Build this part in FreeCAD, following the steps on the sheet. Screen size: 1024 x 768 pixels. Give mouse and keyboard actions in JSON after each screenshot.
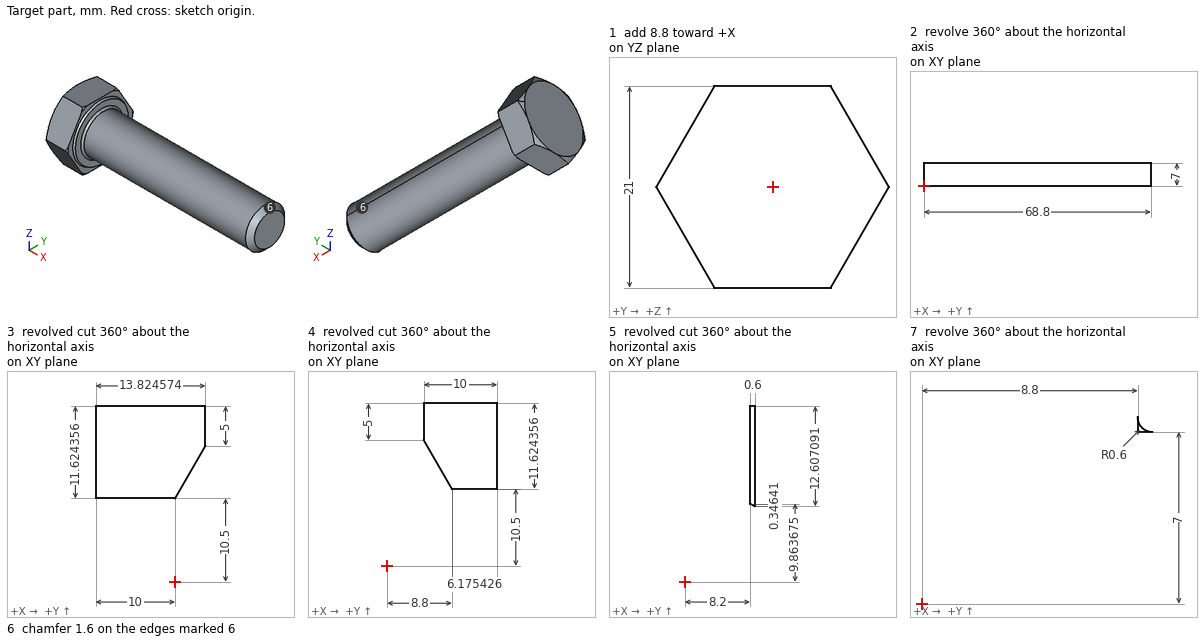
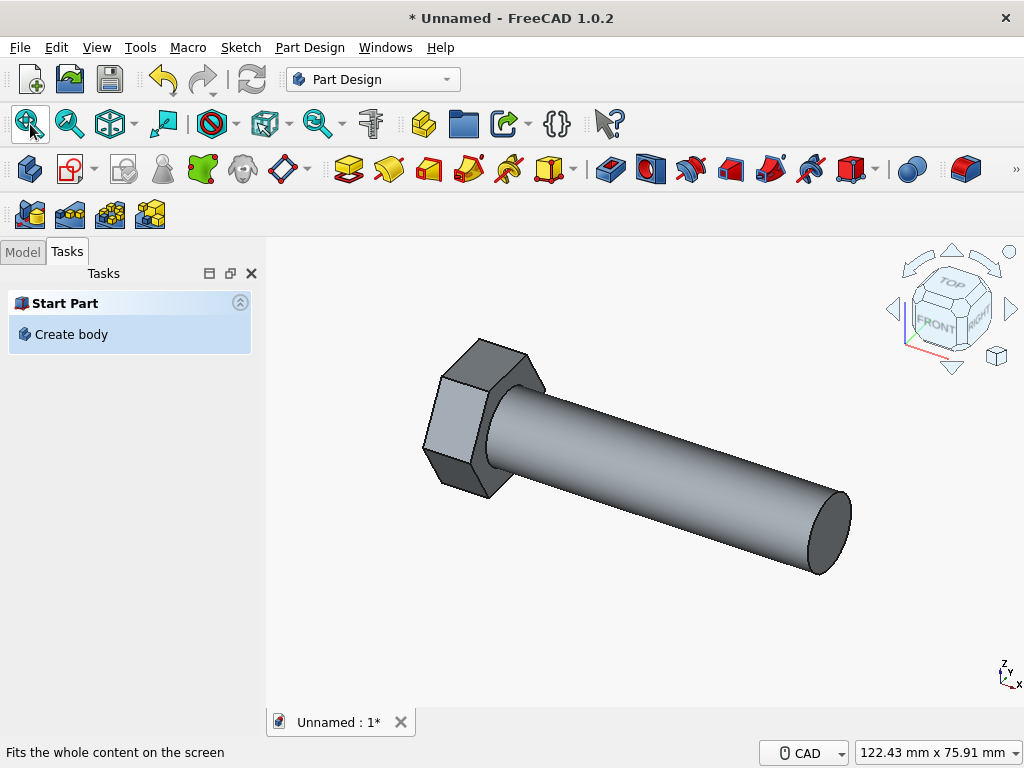
{"action": "left_click", "coordinate": [70, 170]}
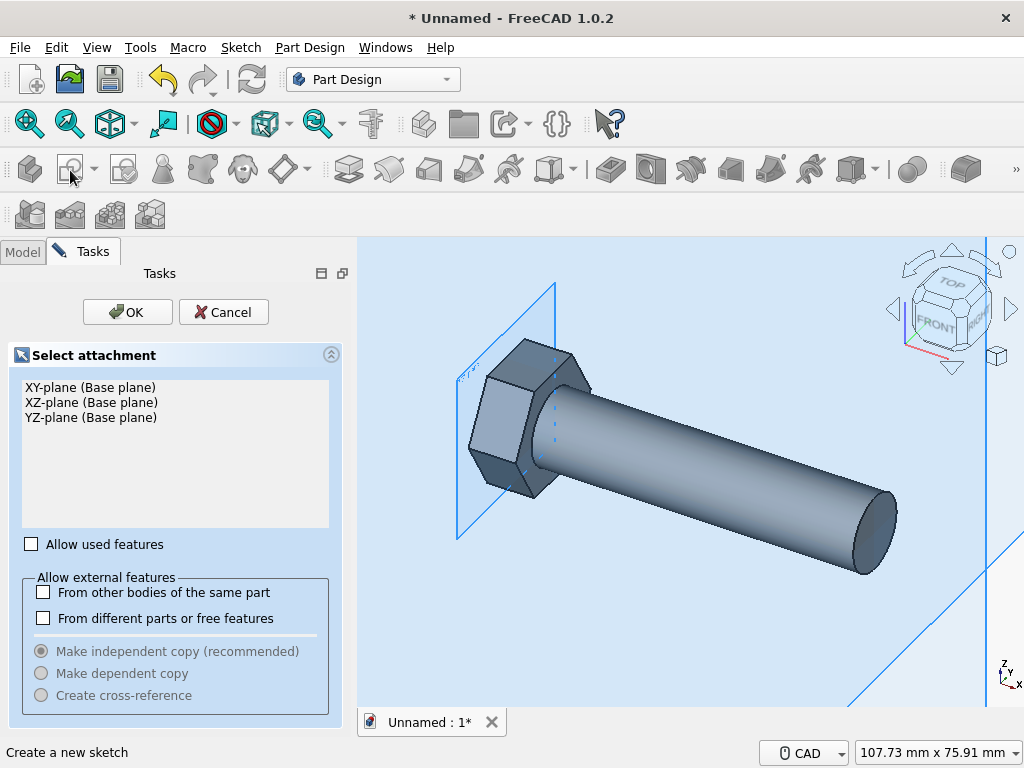
{"action": "left_click", "coordinate": [82, 388]}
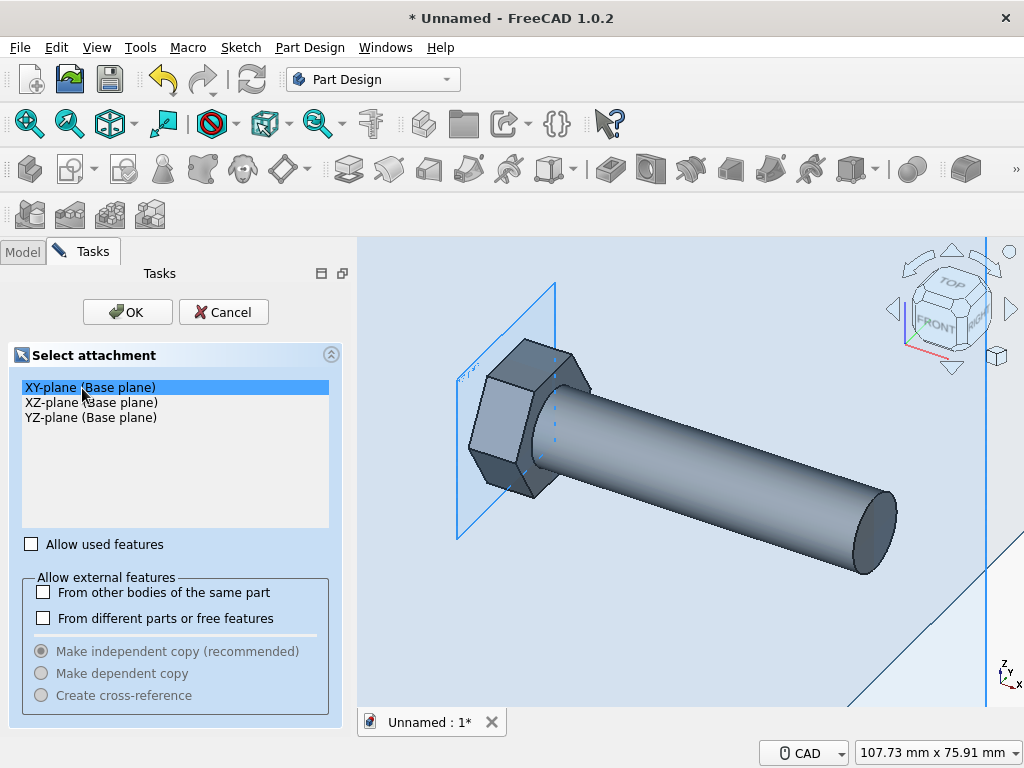
{"action": "left_click", "coordinate": [128, 312]}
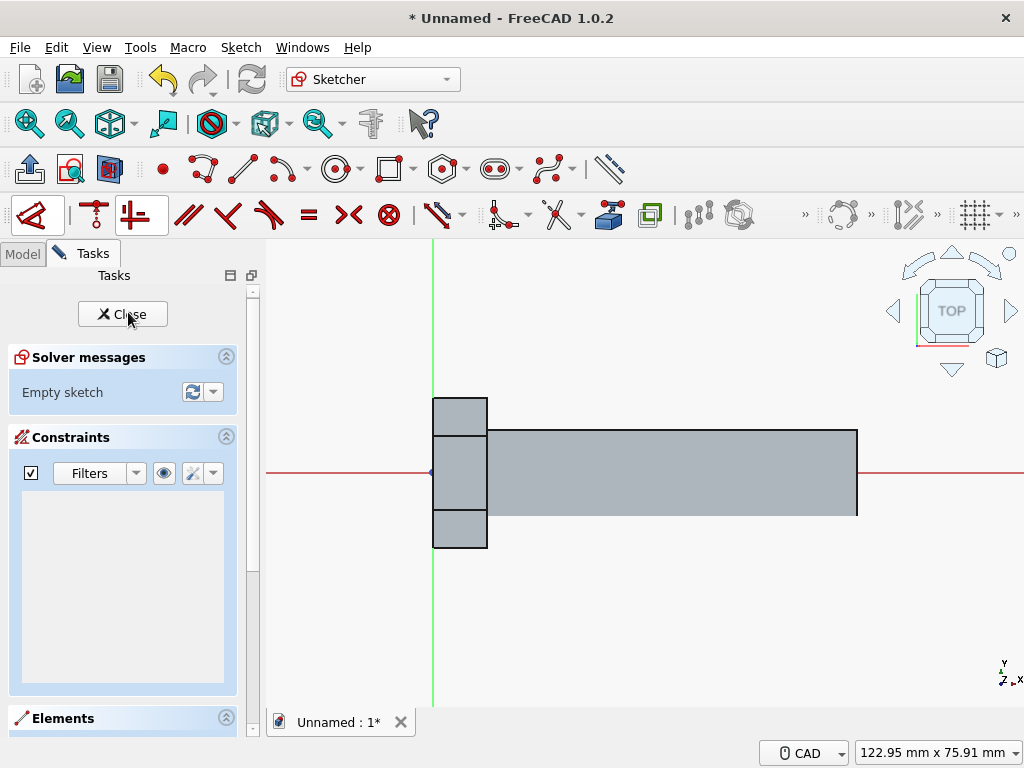
{"action": "left_click", "coordinate": [110, 170]}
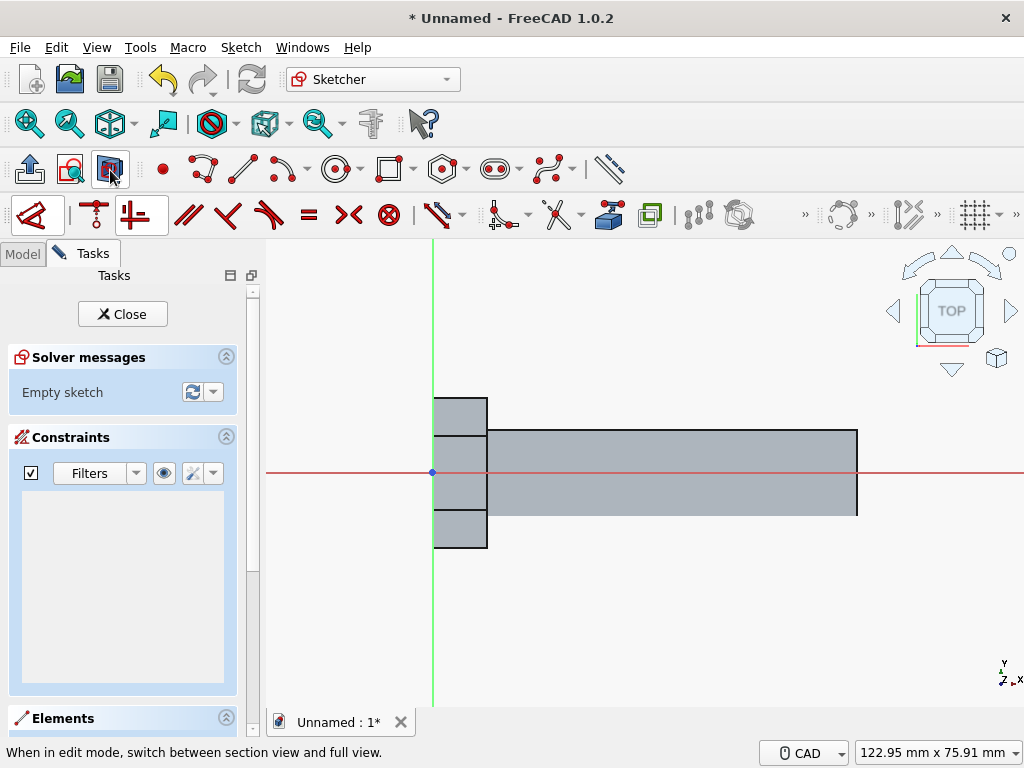
{"action": "scroll", "coordinate": [294, 349], "scroll_direction": "up", "scroll_amount": 4}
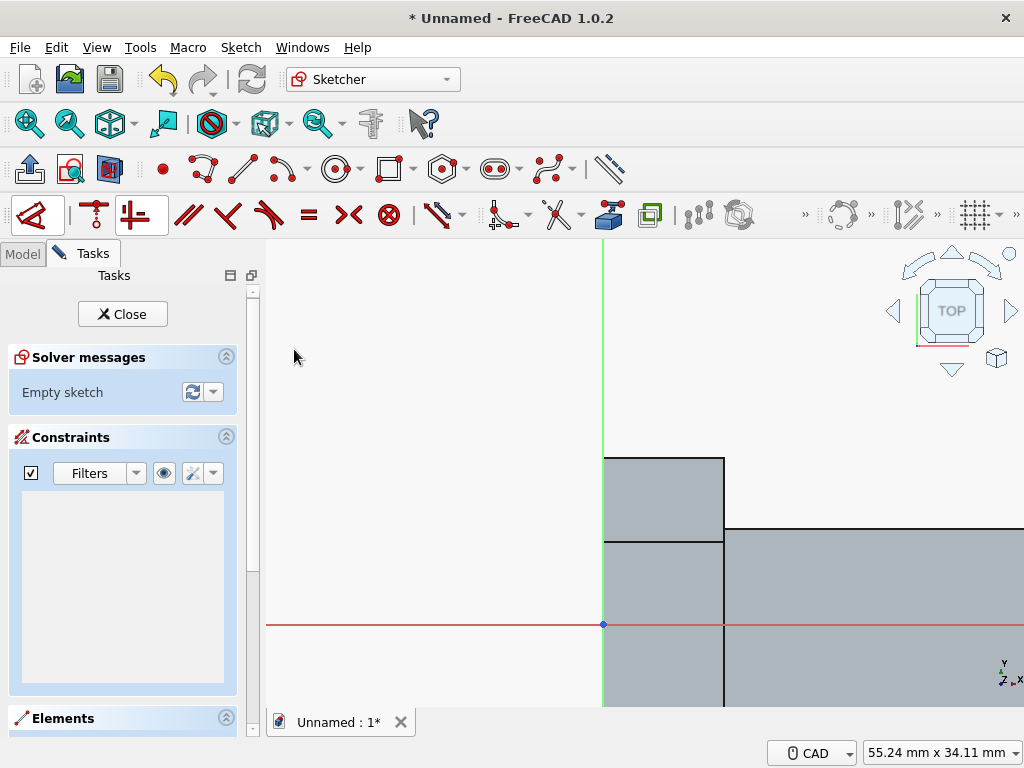
{"action": "left_click", "coordinate": [204, 170]}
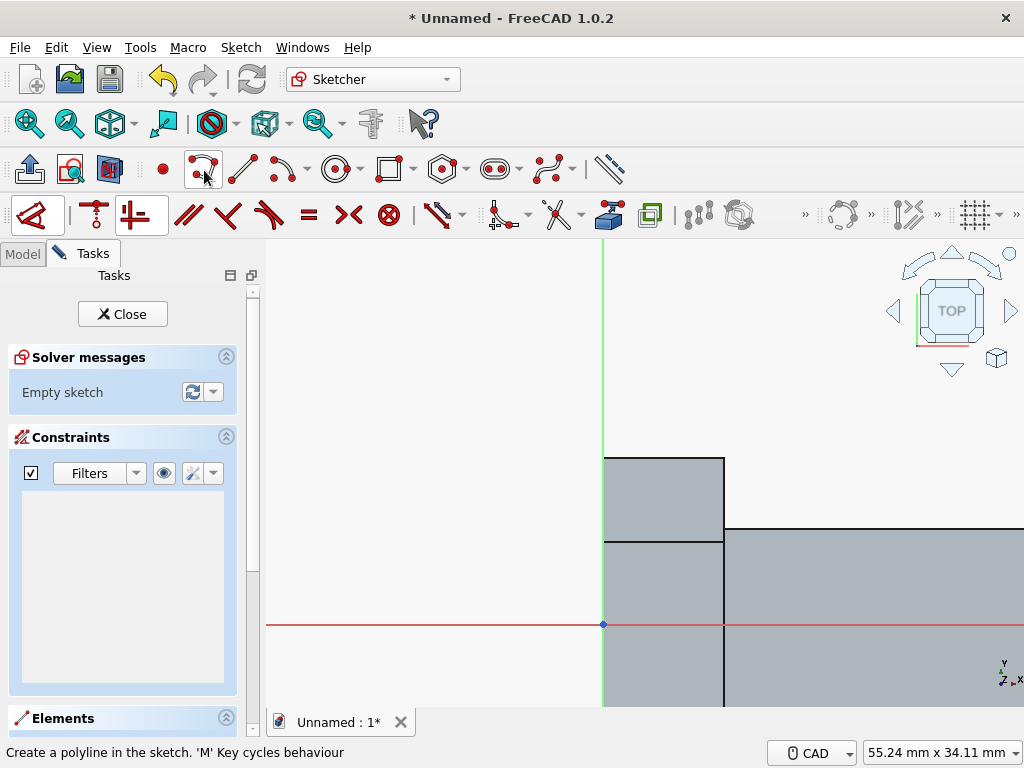
{"action": "left_click", "coordinate": [603, 481]}
{"action": "left_click", "coordinate": [656, 390]}
{"action": "left_click", "coordinate": [656, 321]}
{"action": "left_click", "coordinate": [466, 321]}
{"action": "left_click", "coordinate": [466, 481]}
{"action": "left_click", "coordinate": [603, 482]}
{"action": "key", "text": "Escape"}
{"action": "key", "text": "Escape"}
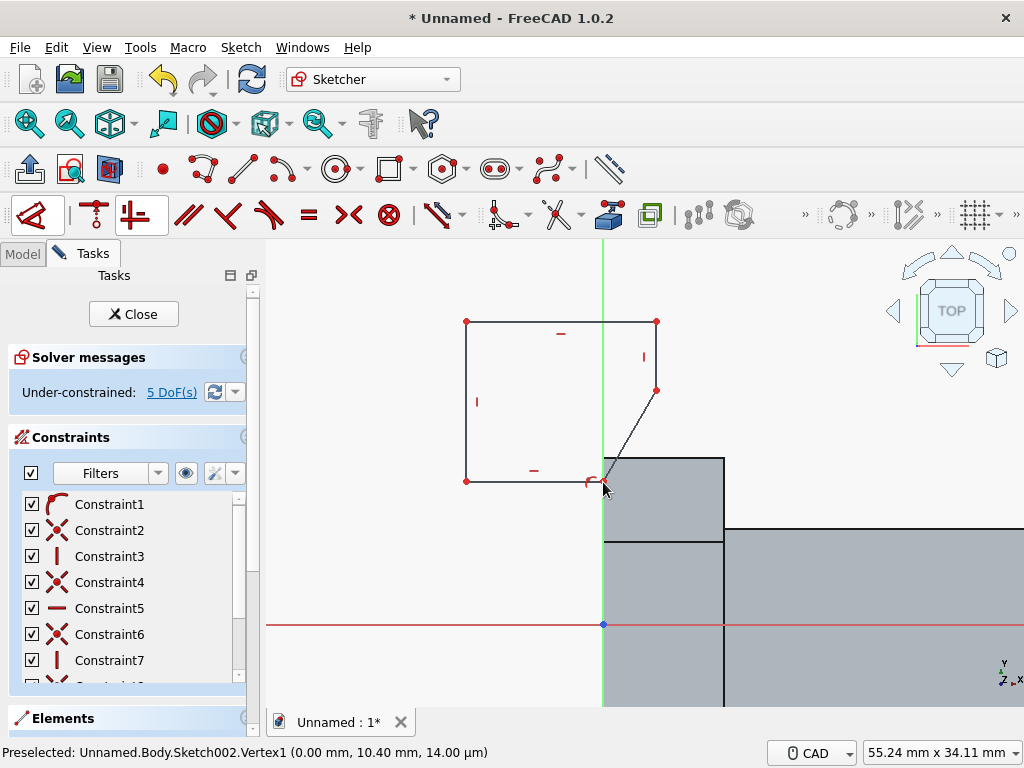
{"action": "left_click", "coordinate": [656, 370]}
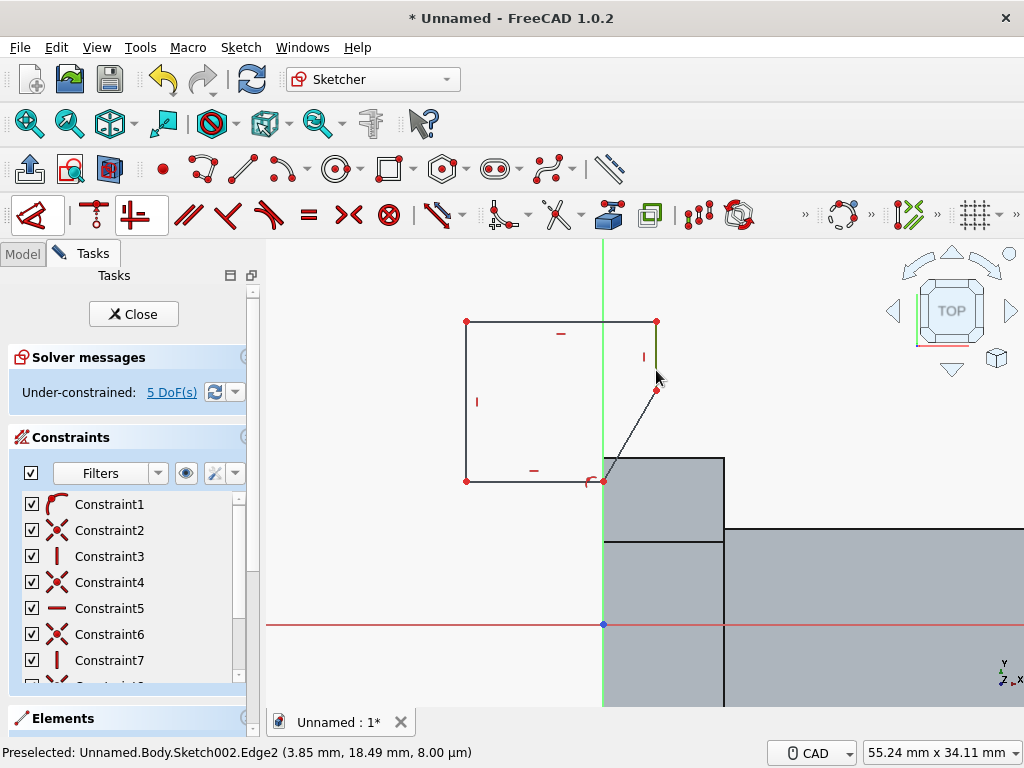
{"action": "left_click", "coordinate": [58, 216]}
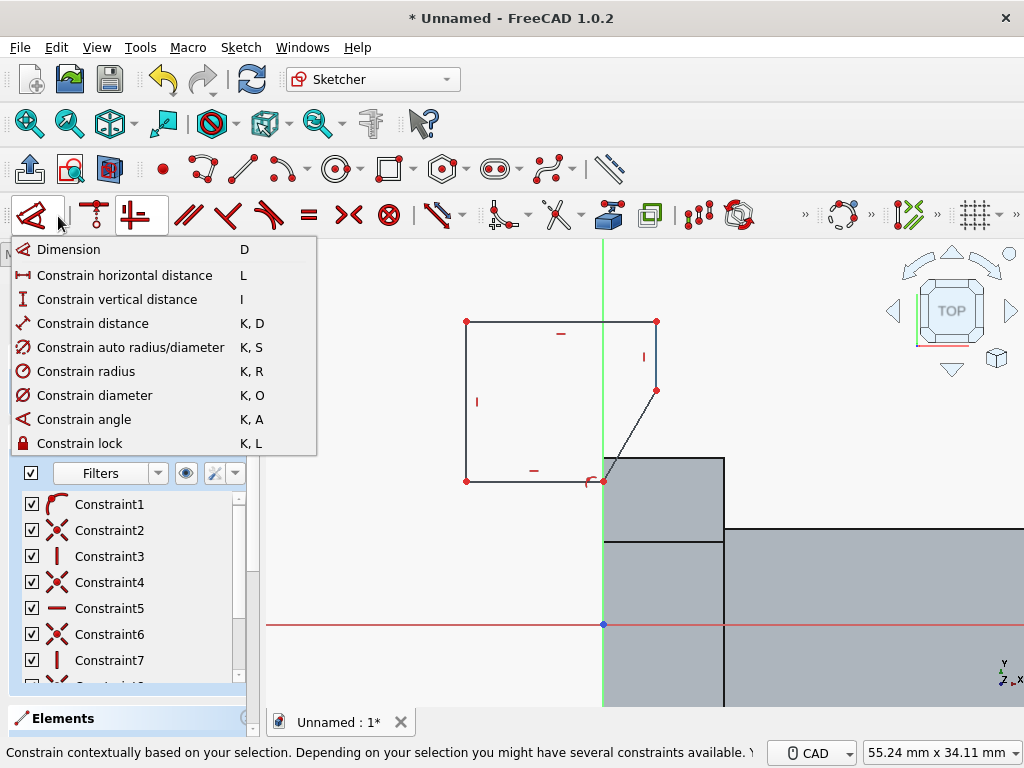
{"action": "left_click", "coordinate": [164, 299]}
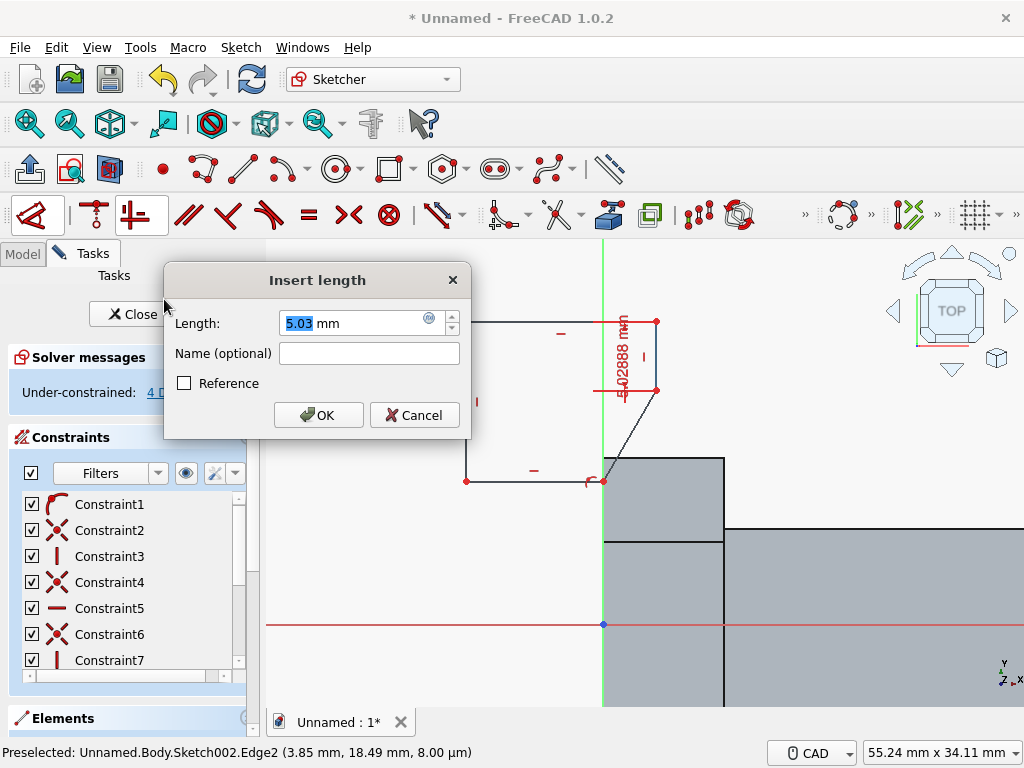
{"action": "type", "text": "5"}
{"action": "key", "text": "Return"}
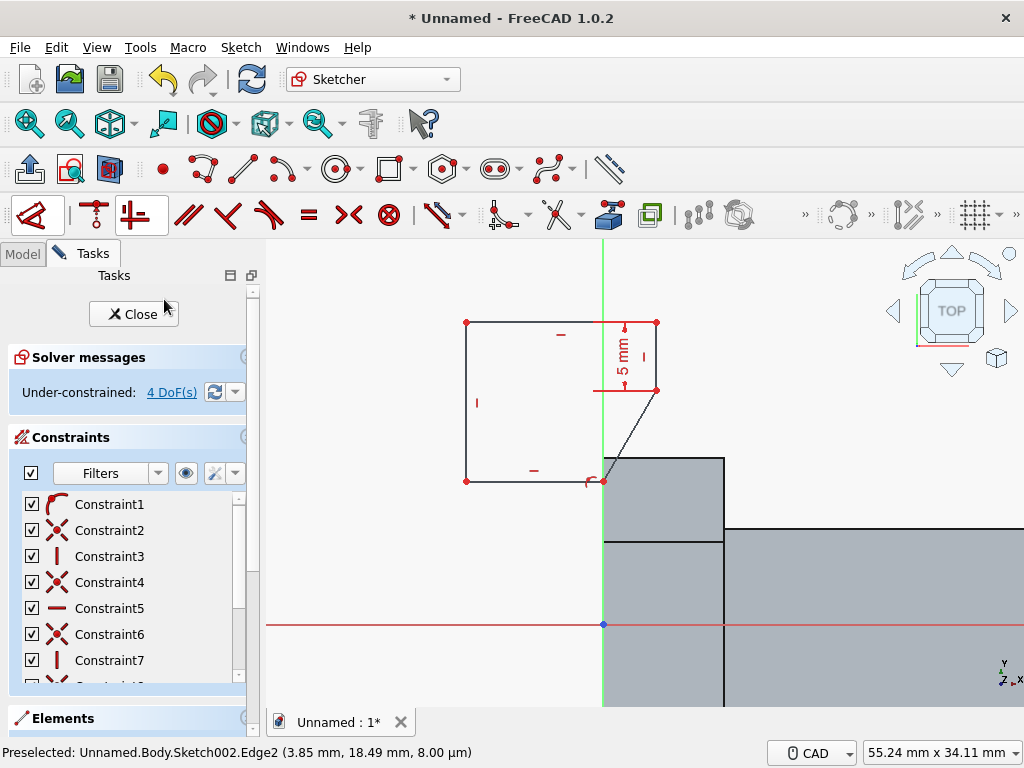
{"action": "left_click", "coordinate": [507, 482]}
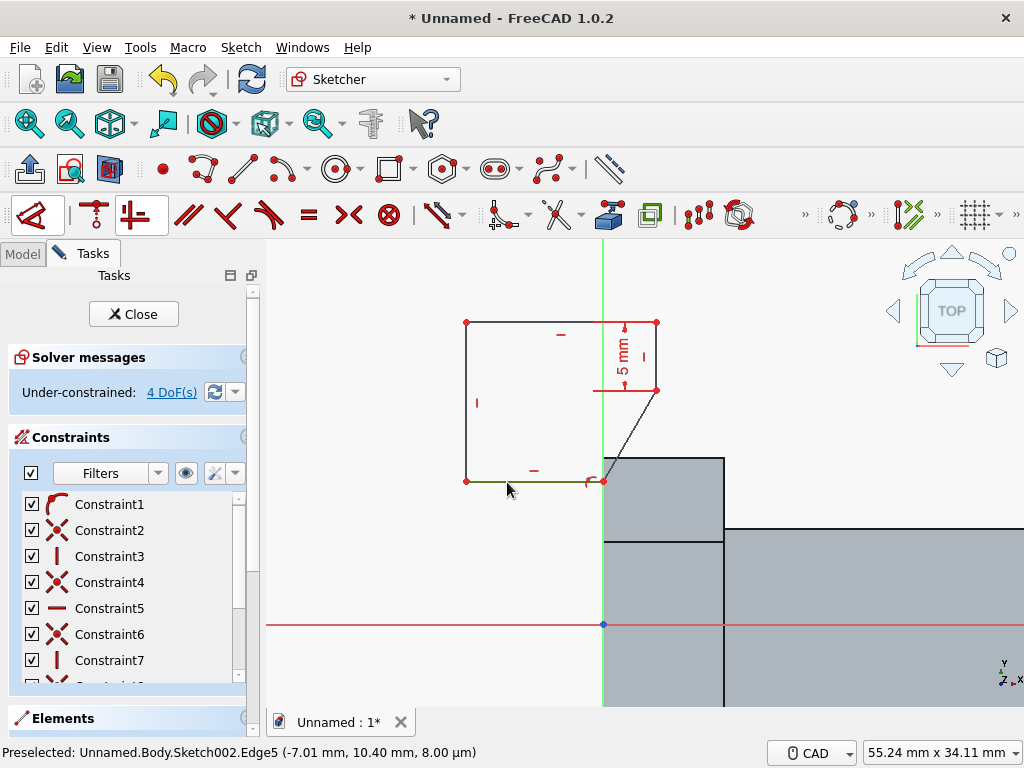
{"action": "key", "text": "l"}